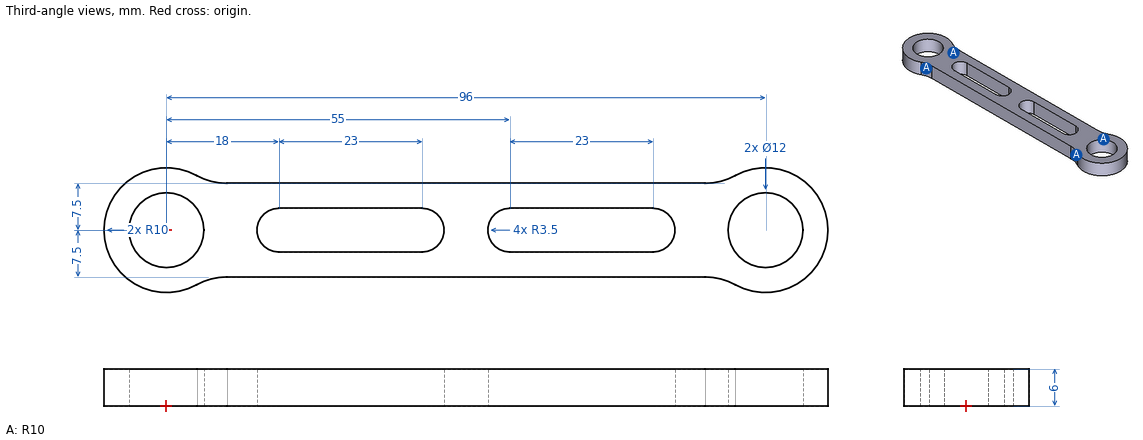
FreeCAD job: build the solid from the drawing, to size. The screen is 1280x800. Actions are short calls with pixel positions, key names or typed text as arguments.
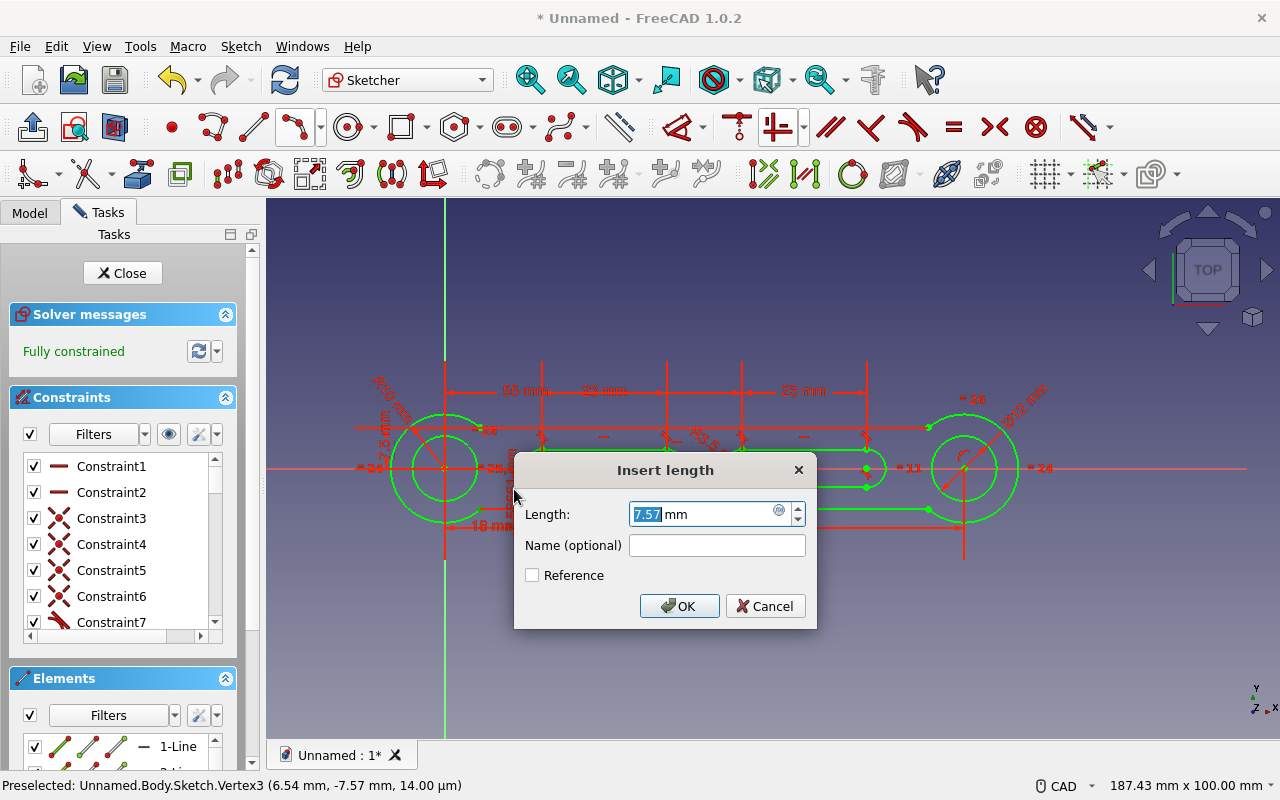
text(7.5)
key(Return)
key(Escape)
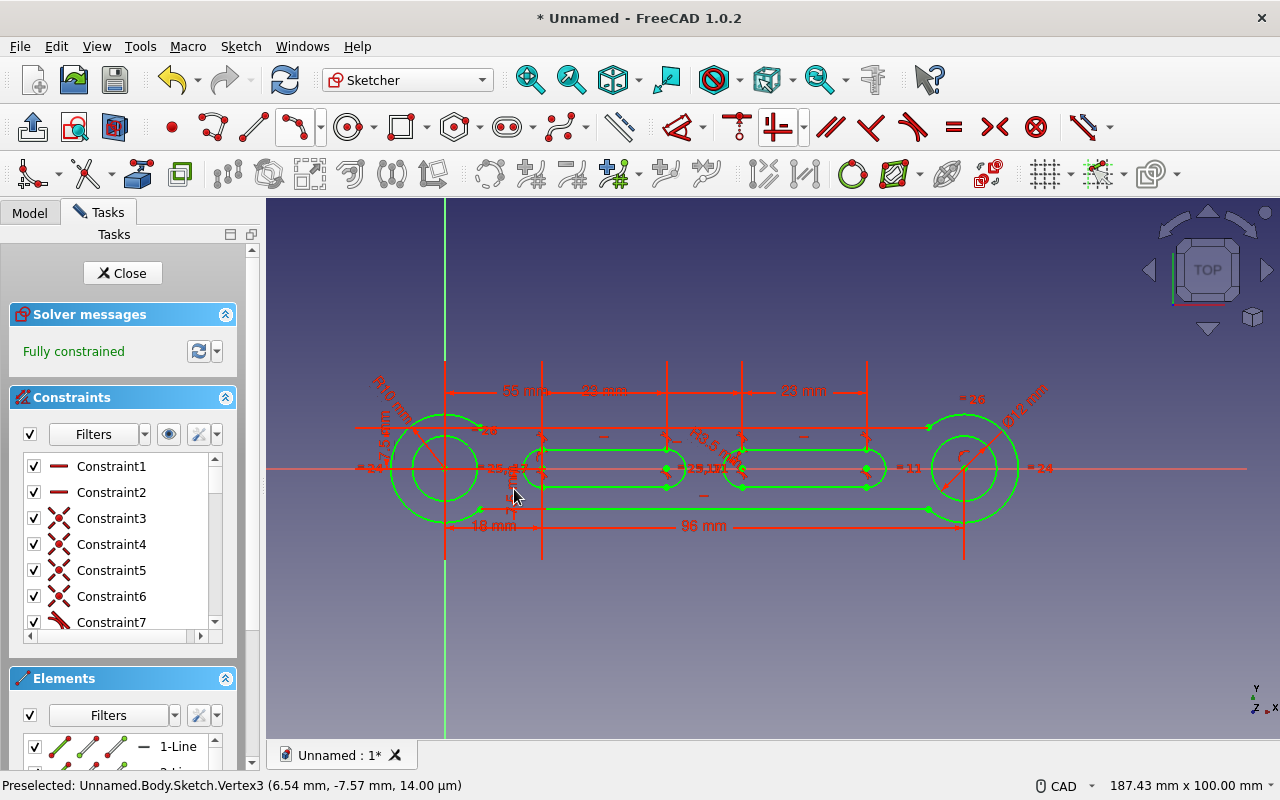
click(123, 273)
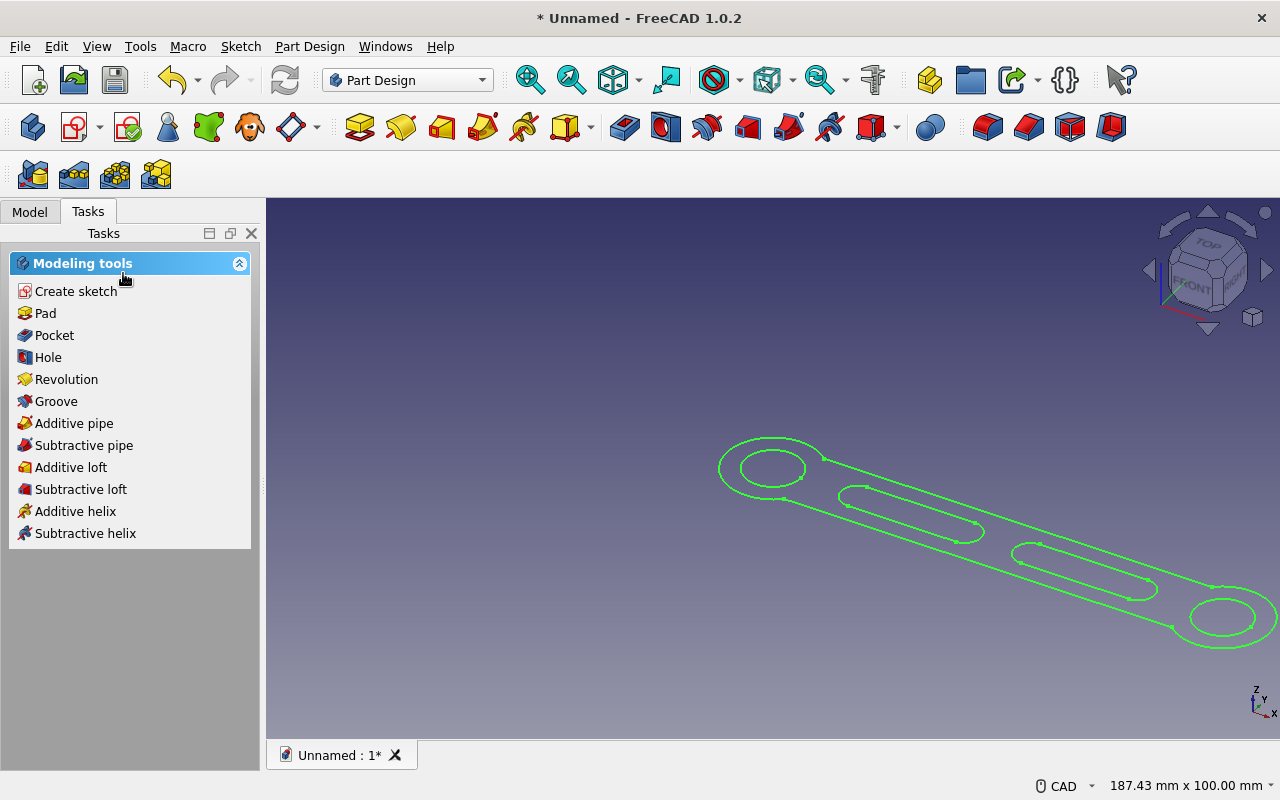
click(360, 128)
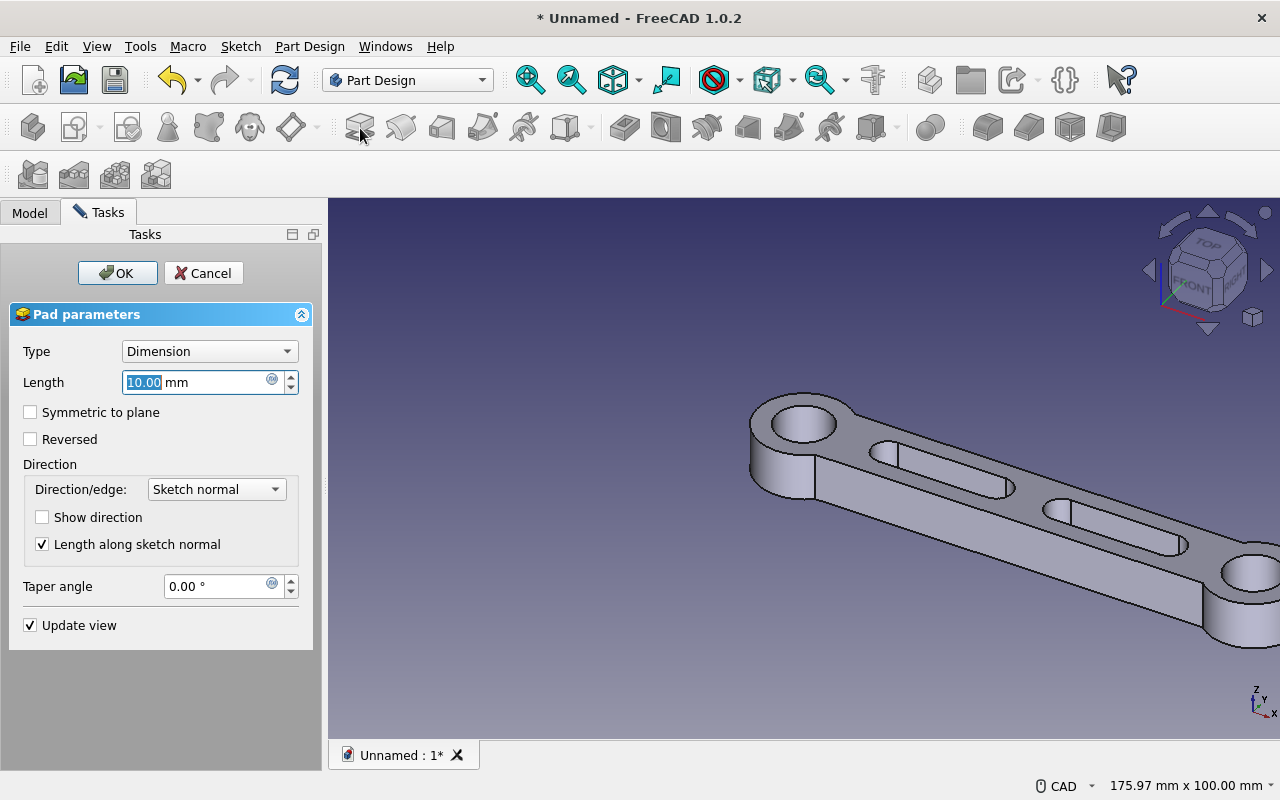
text(6)
key(Tab)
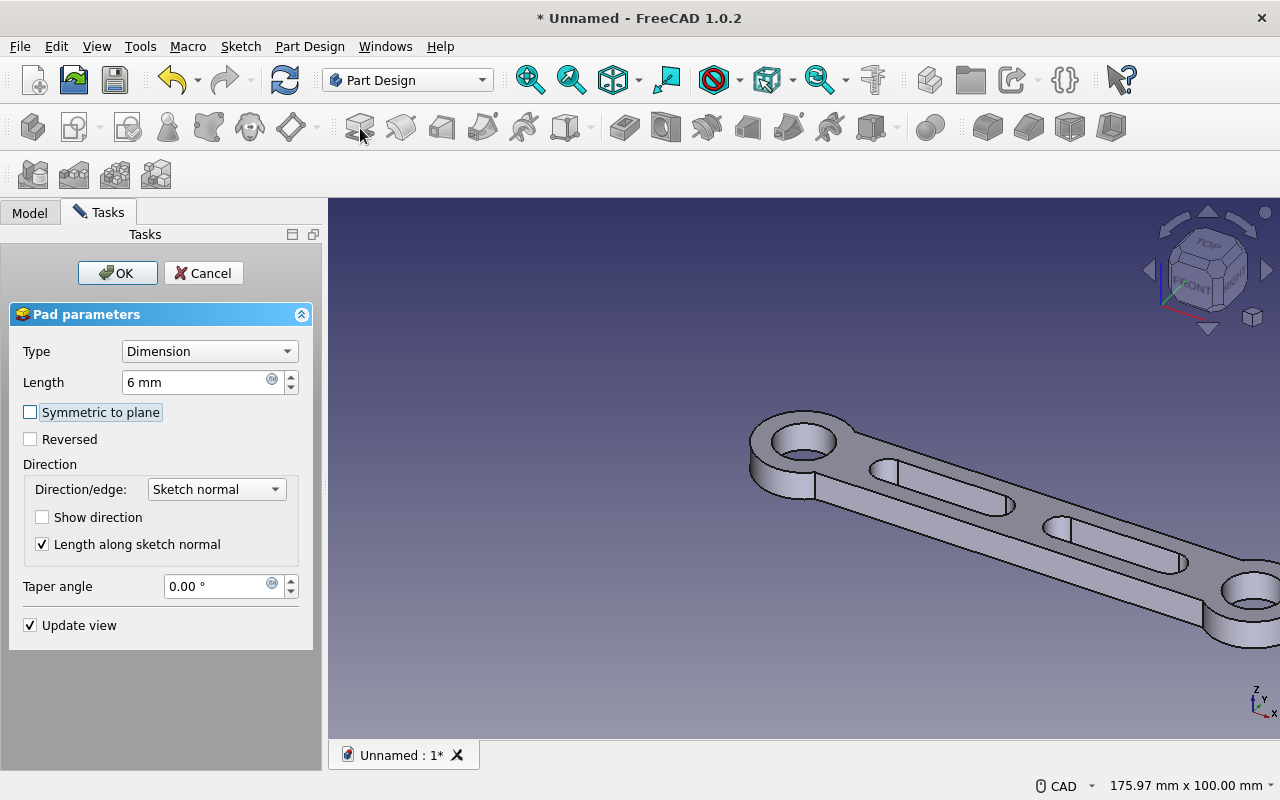
click(118, 273)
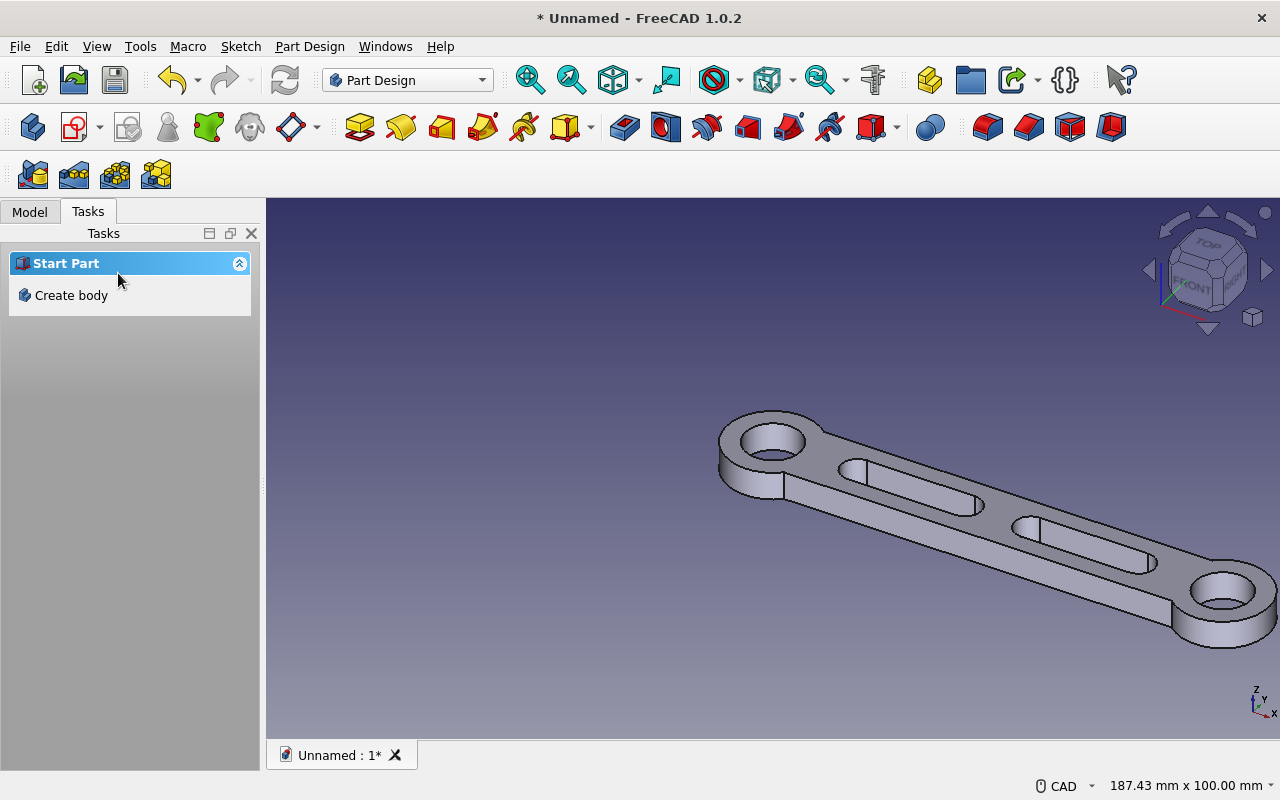
click(531, 80)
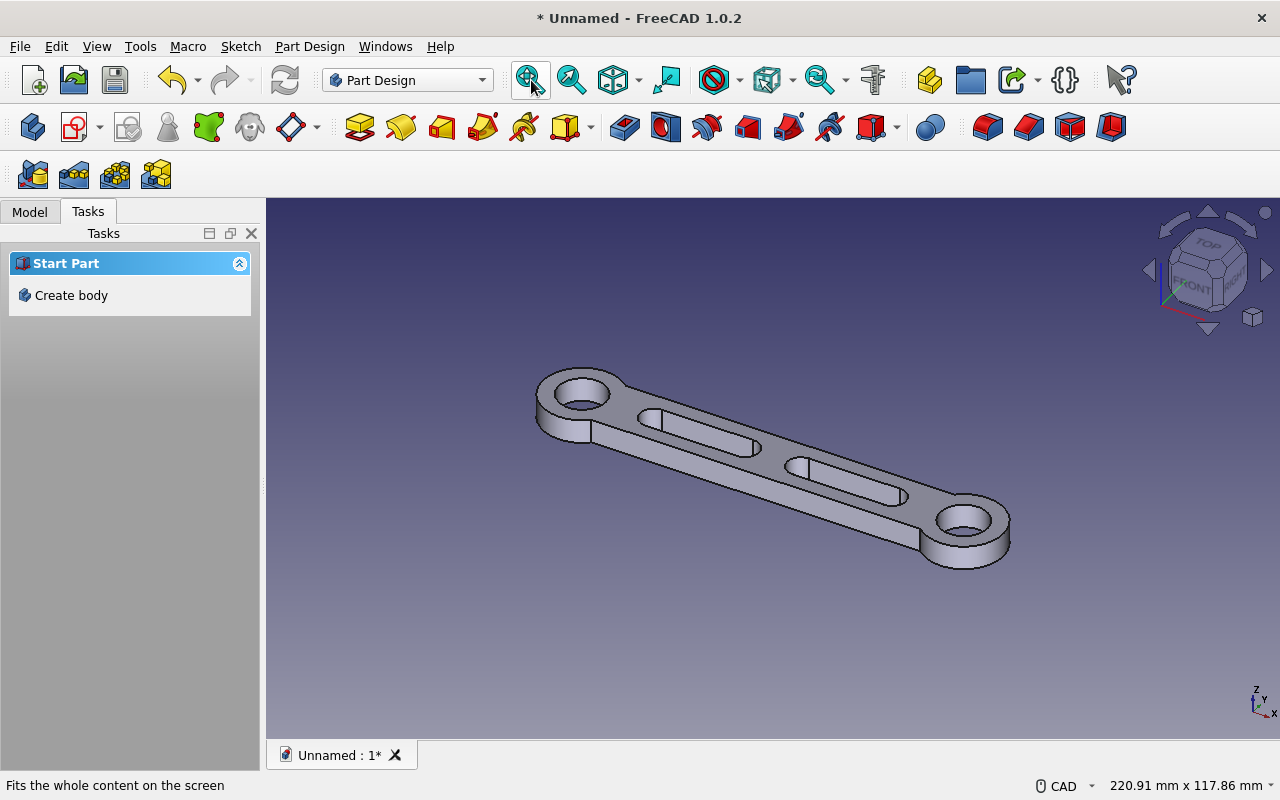
key(0)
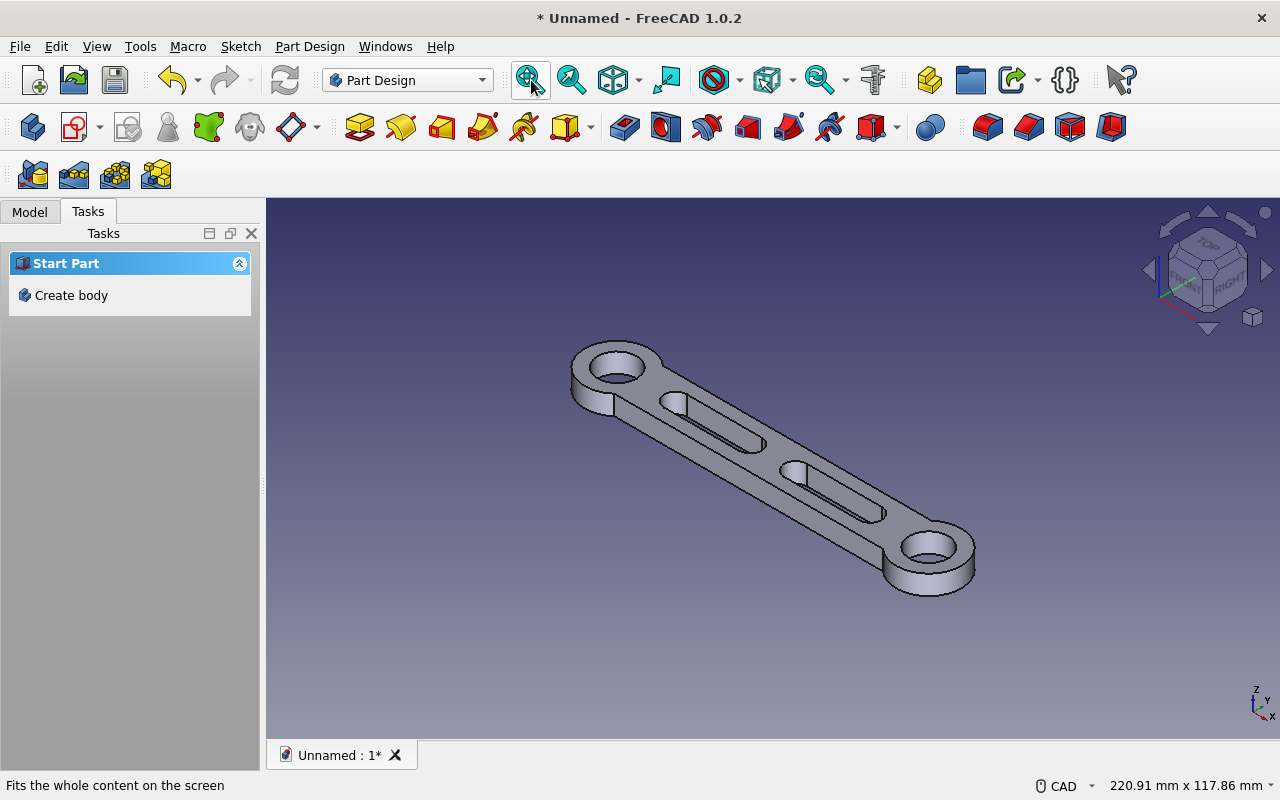
key(2)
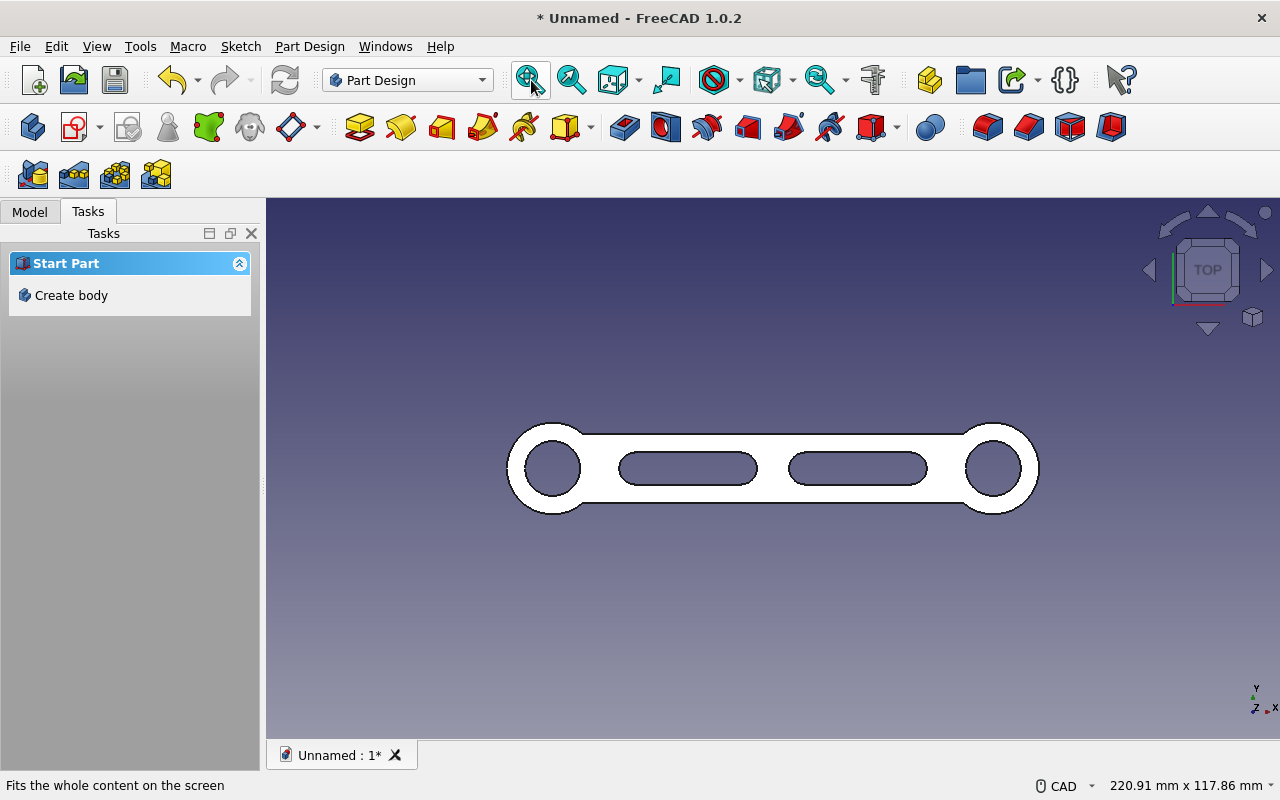
key(1)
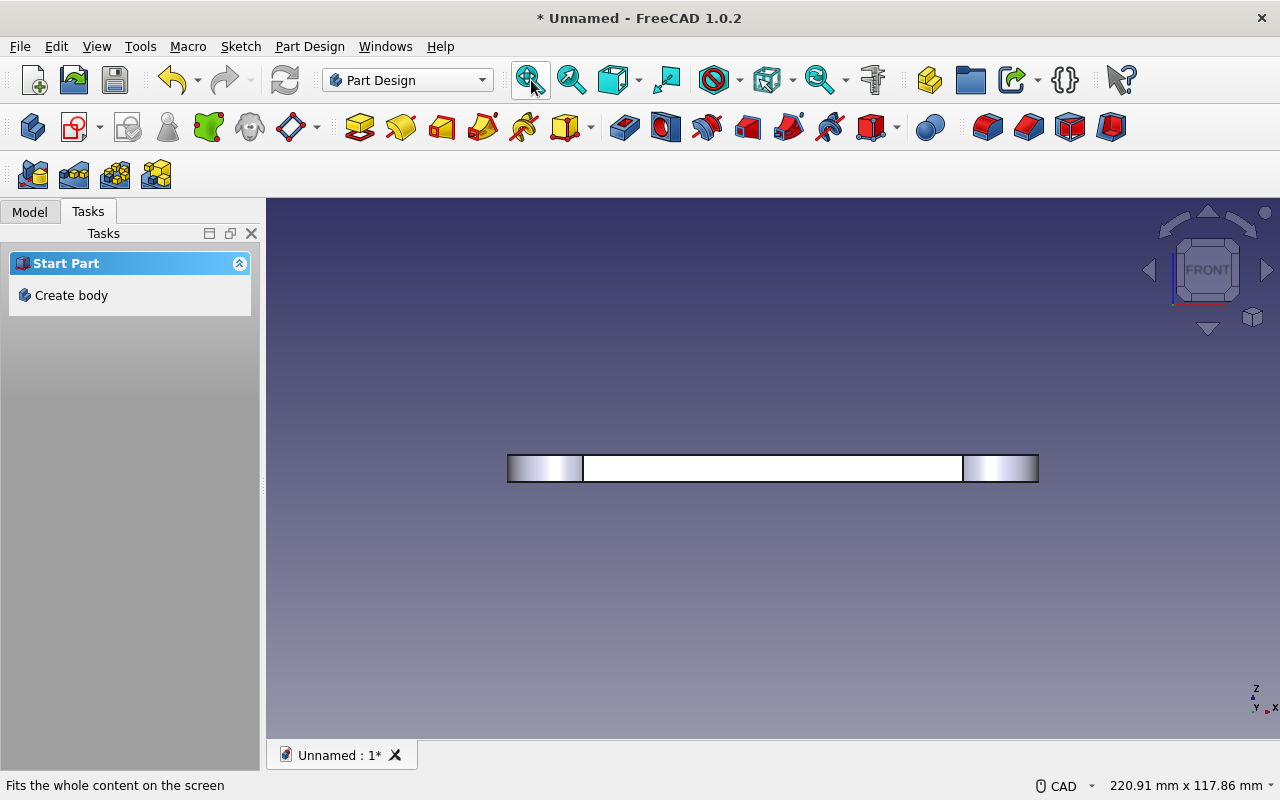
key(3)